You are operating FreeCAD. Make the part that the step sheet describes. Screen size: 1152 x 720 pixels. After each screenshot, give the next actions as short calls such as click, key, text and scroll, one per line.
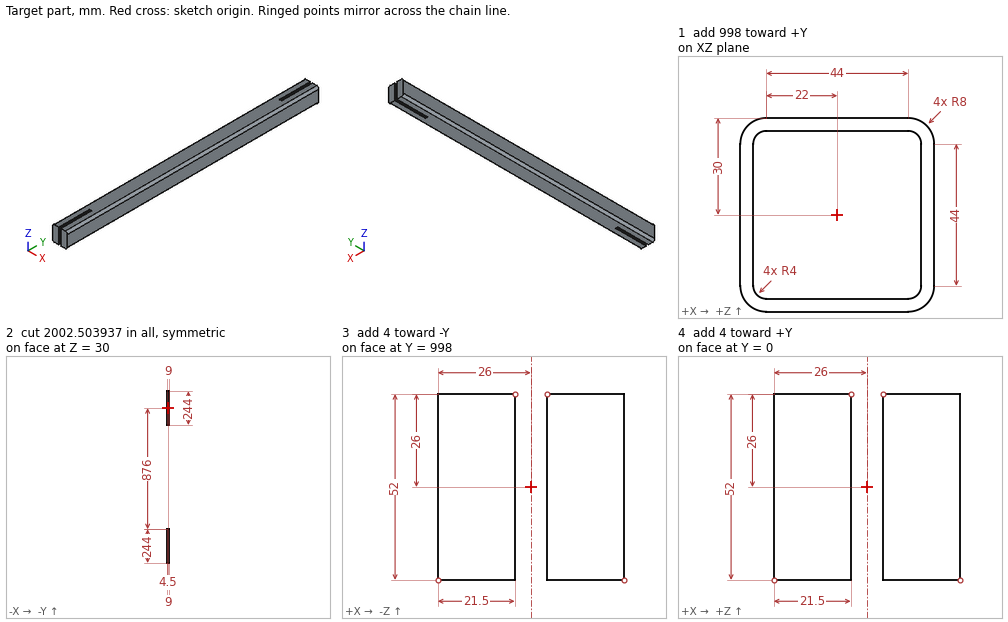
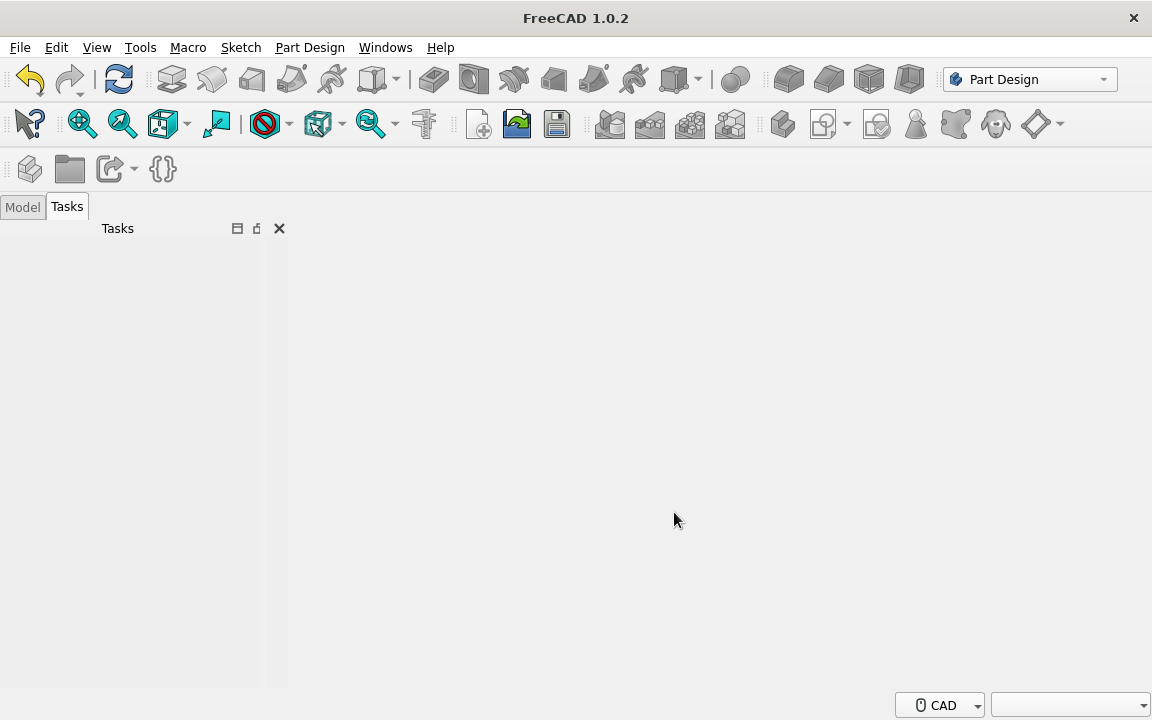
click(478, 124)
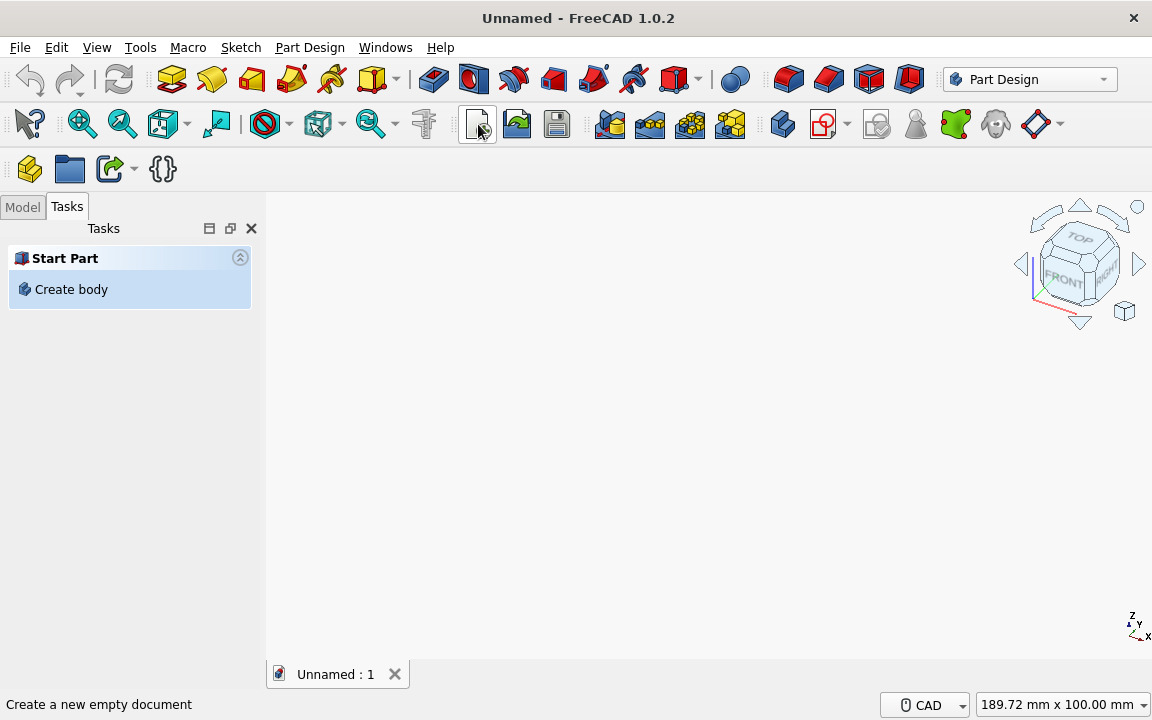
click(824, 124)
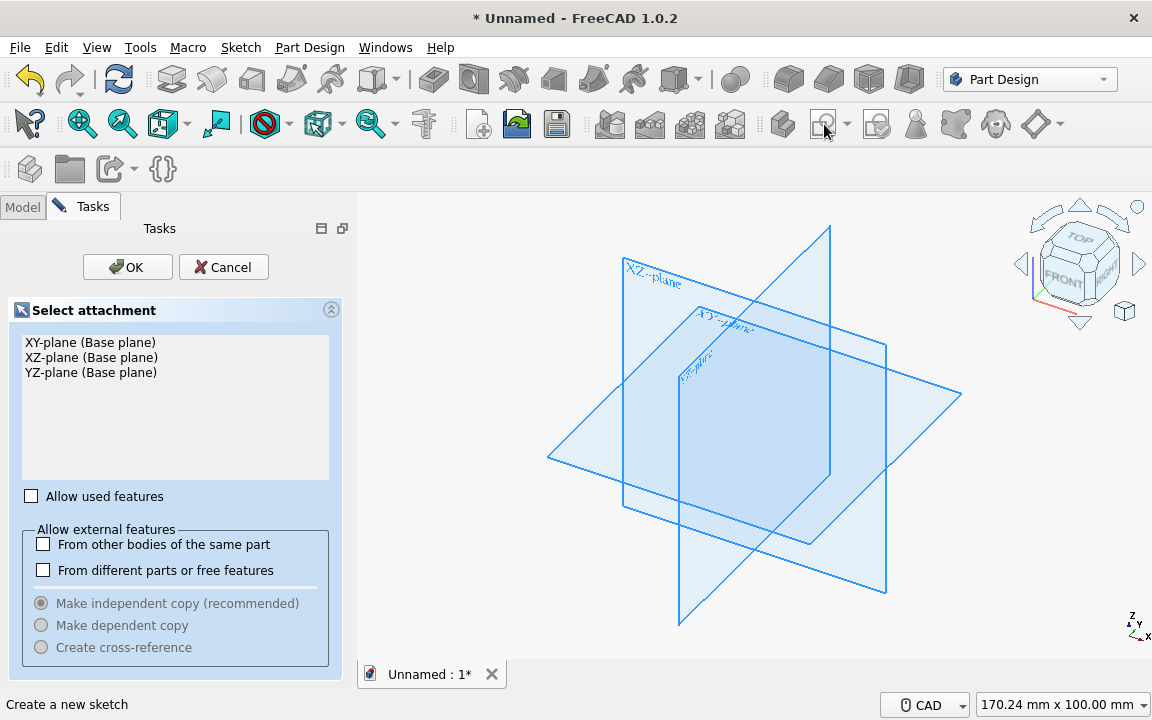
click(82, 358)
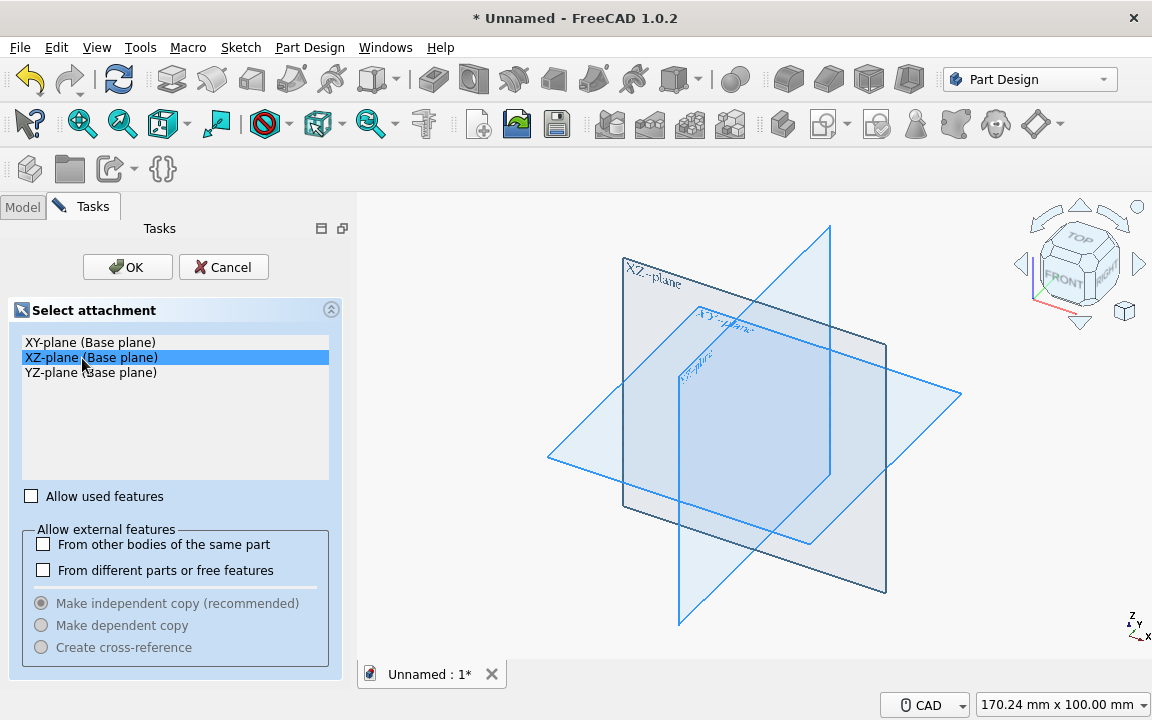
click(128, 267)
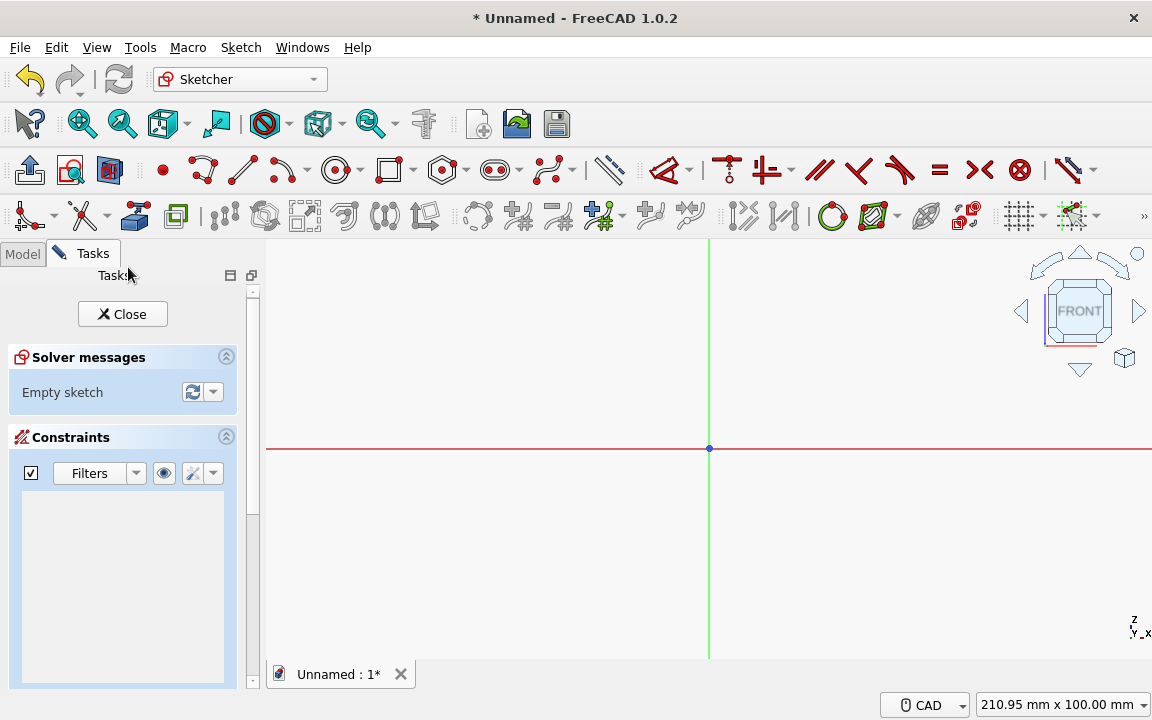
click(244, 170)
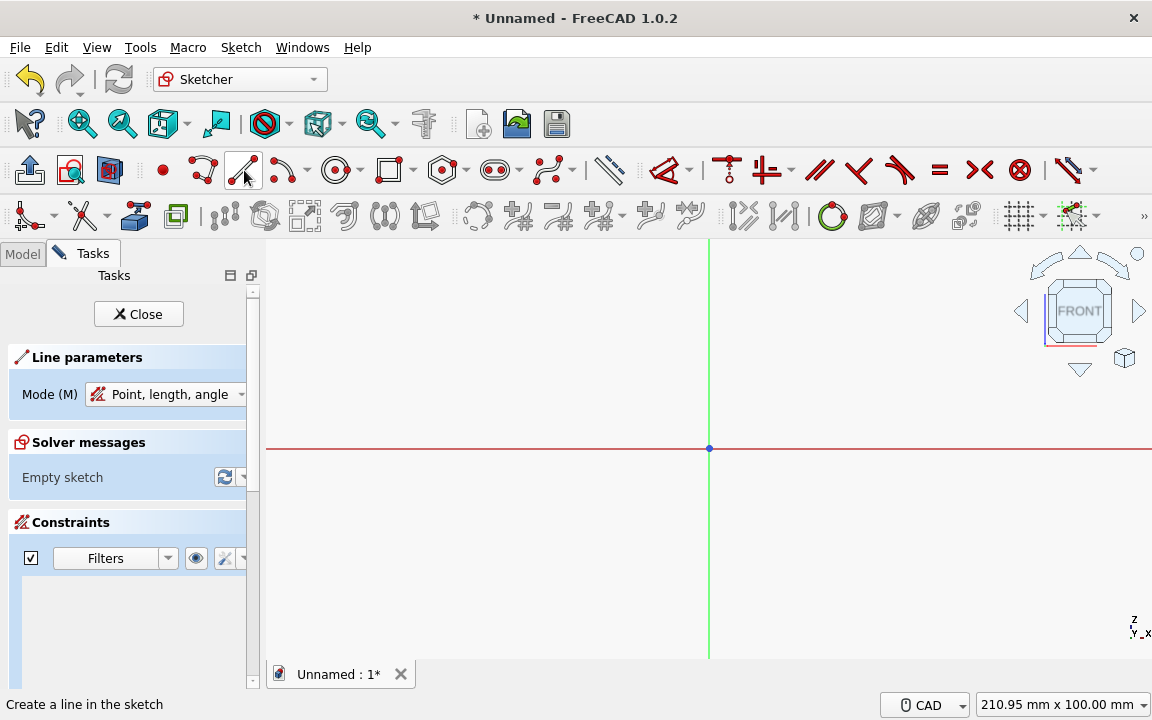
click(617, 323)
click(801, 323)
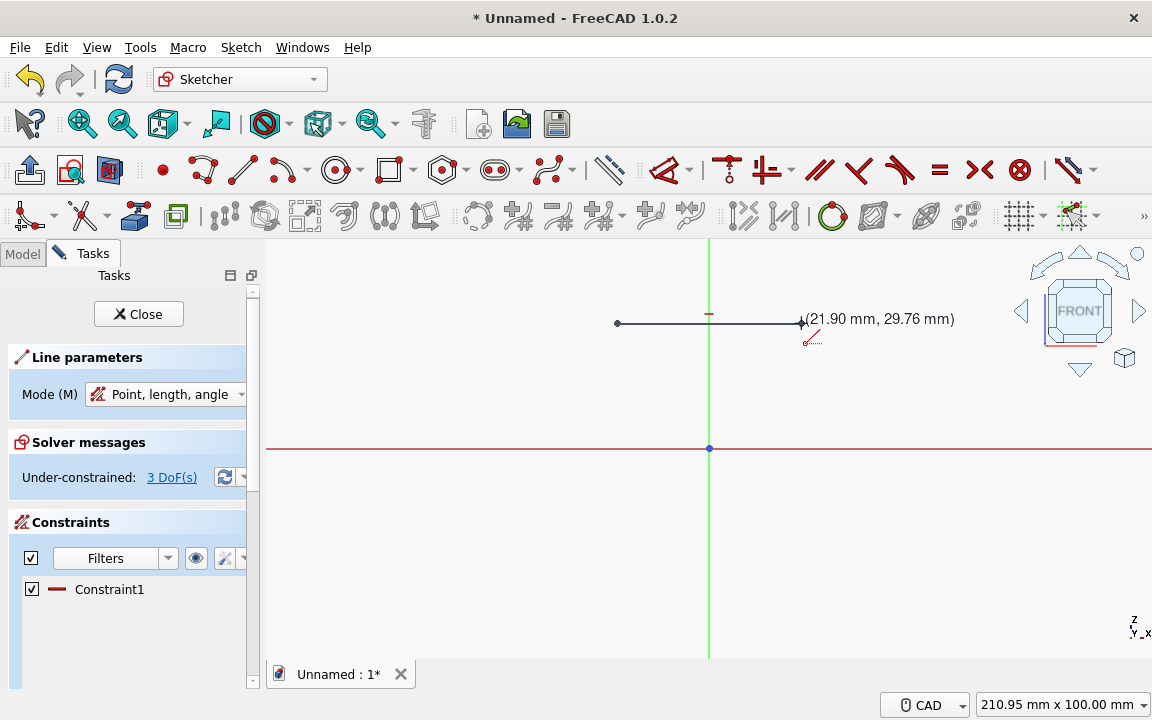
click(835, 357)
click(835, 541)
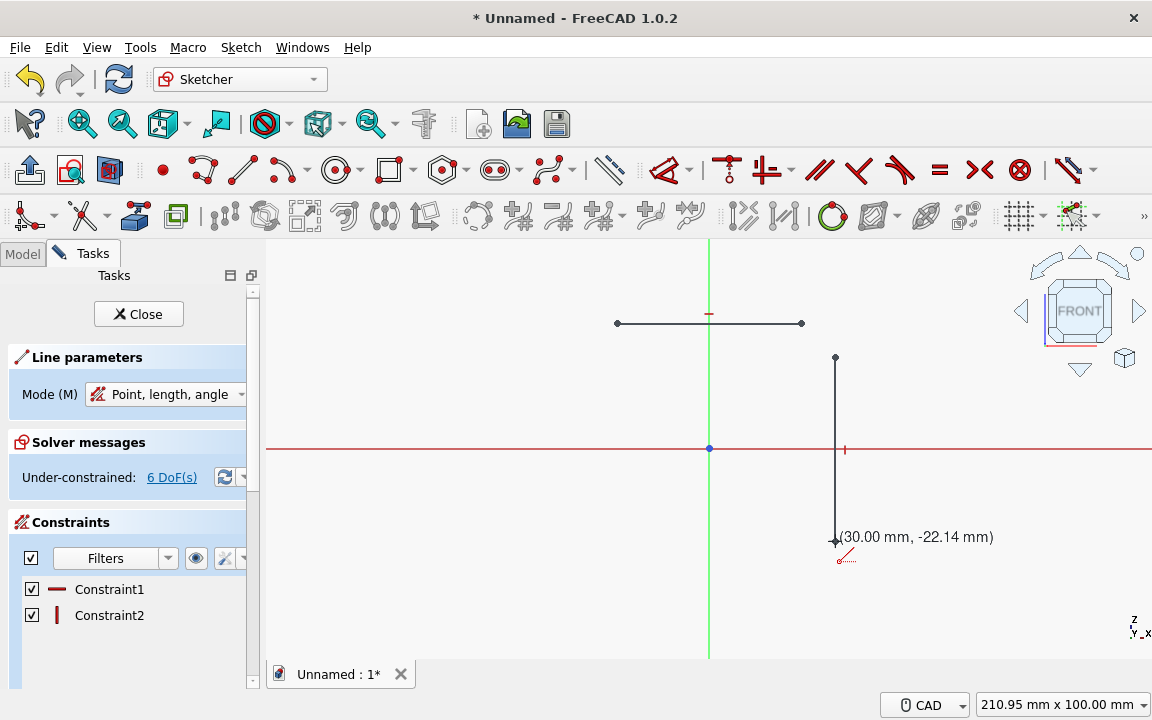
click(801, 575)
click(617, 575)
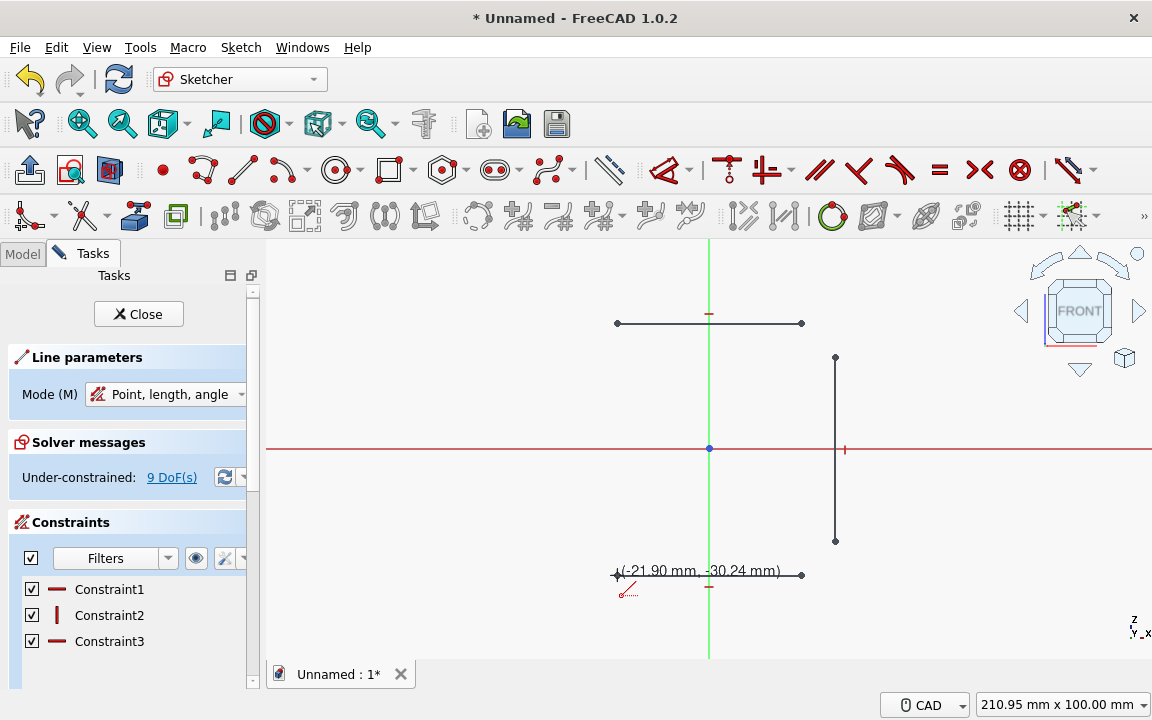
click(583, 541)
click(583, 357)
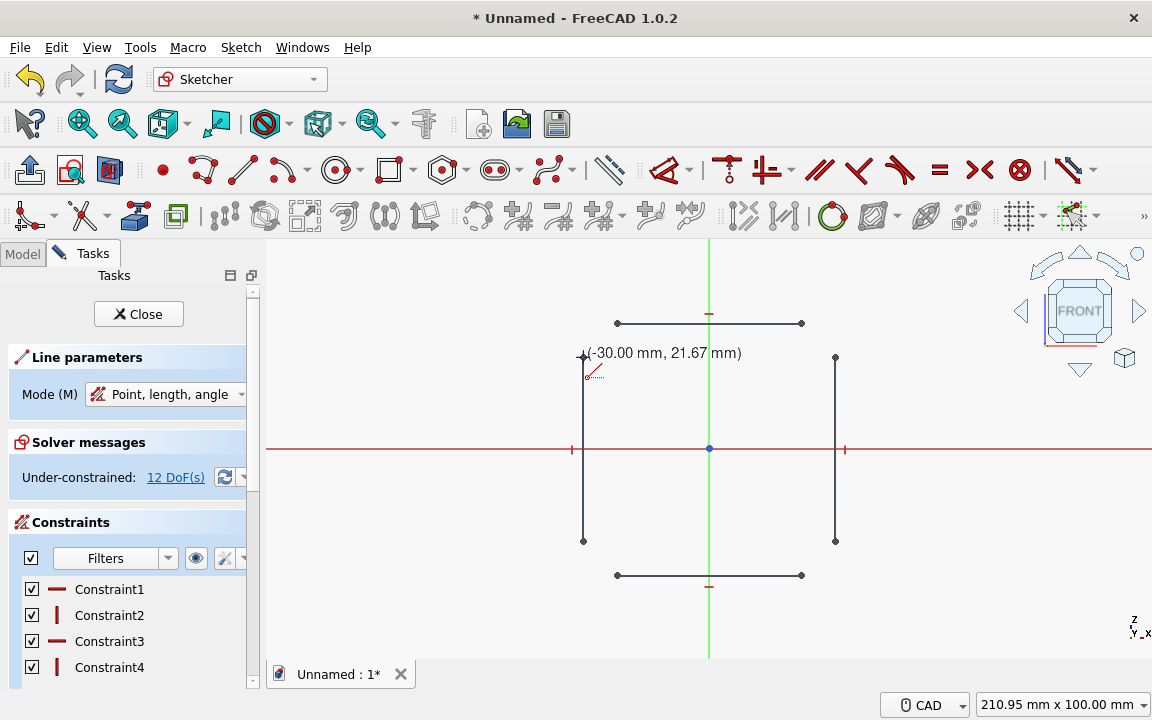
key(g)
key(3)
key(a)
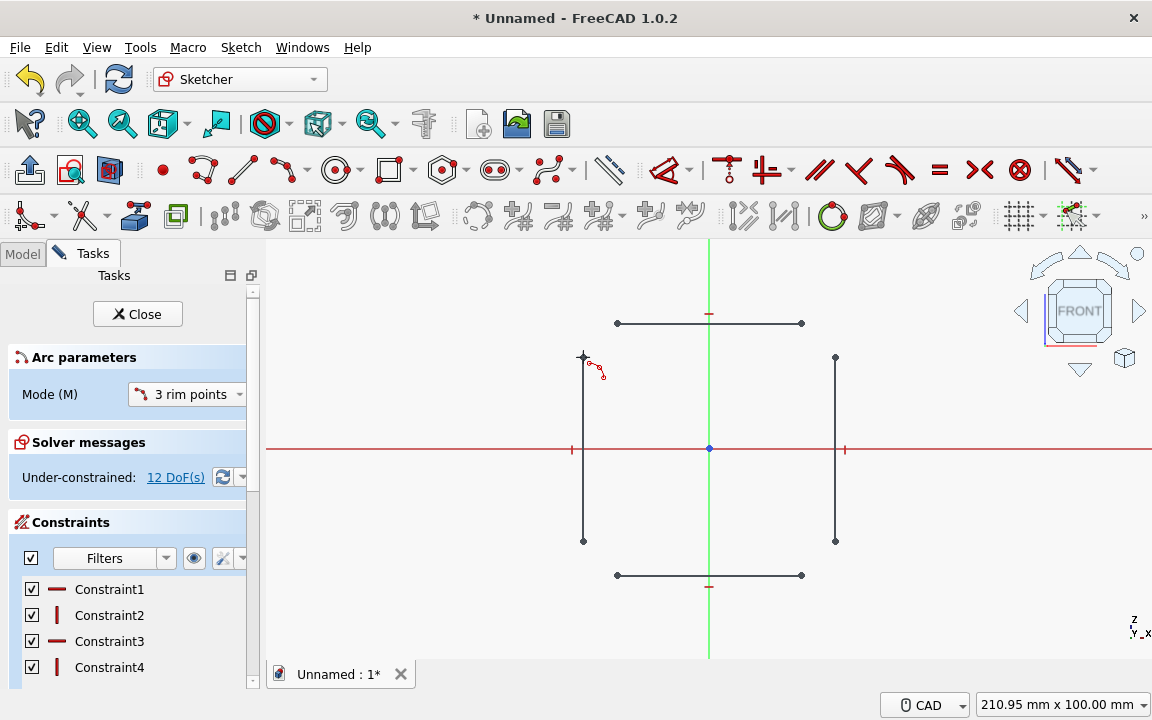
click(801, 324)
click(835, 358)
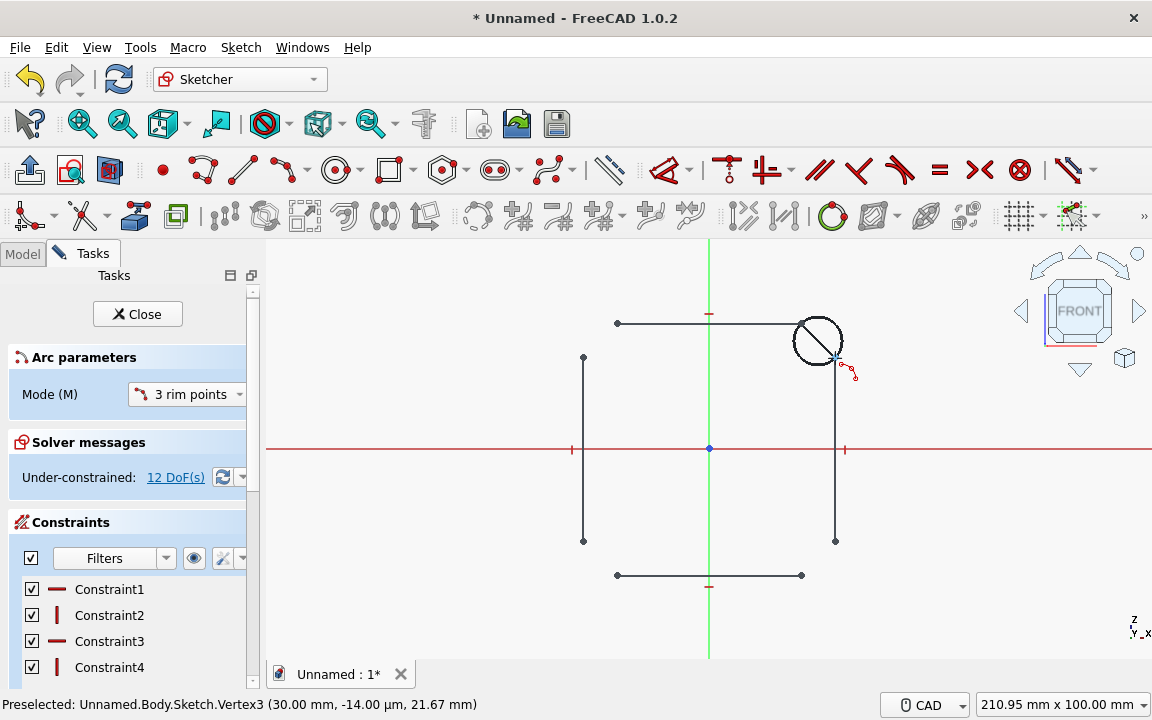
scroll(825, 333, up, 3)